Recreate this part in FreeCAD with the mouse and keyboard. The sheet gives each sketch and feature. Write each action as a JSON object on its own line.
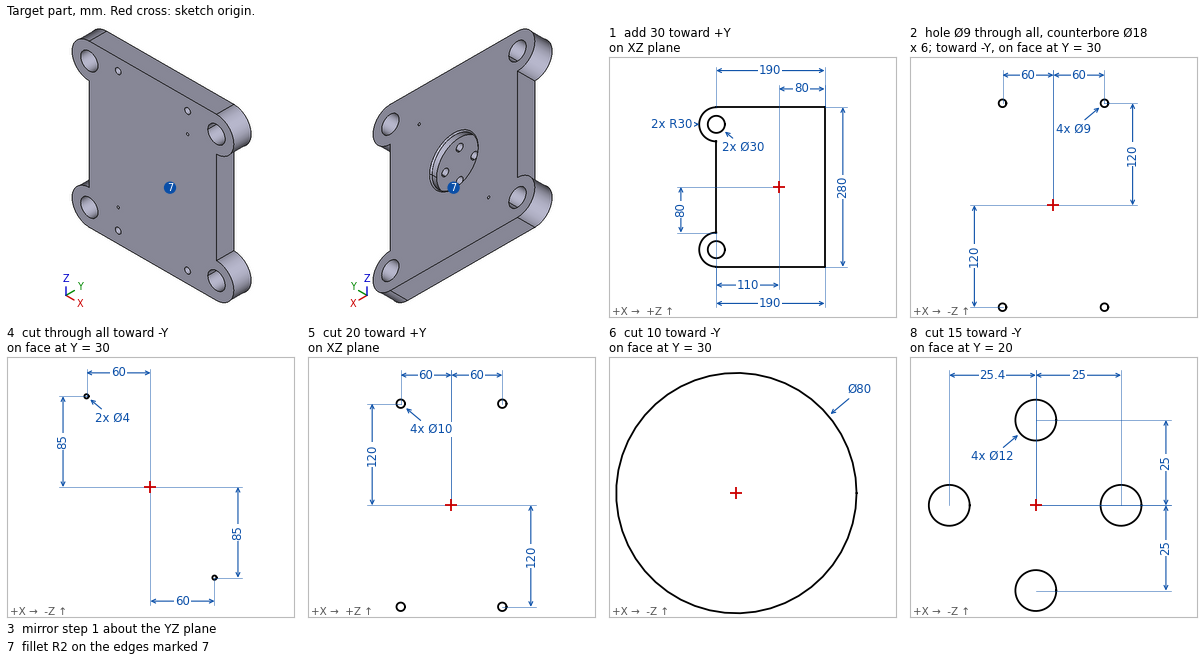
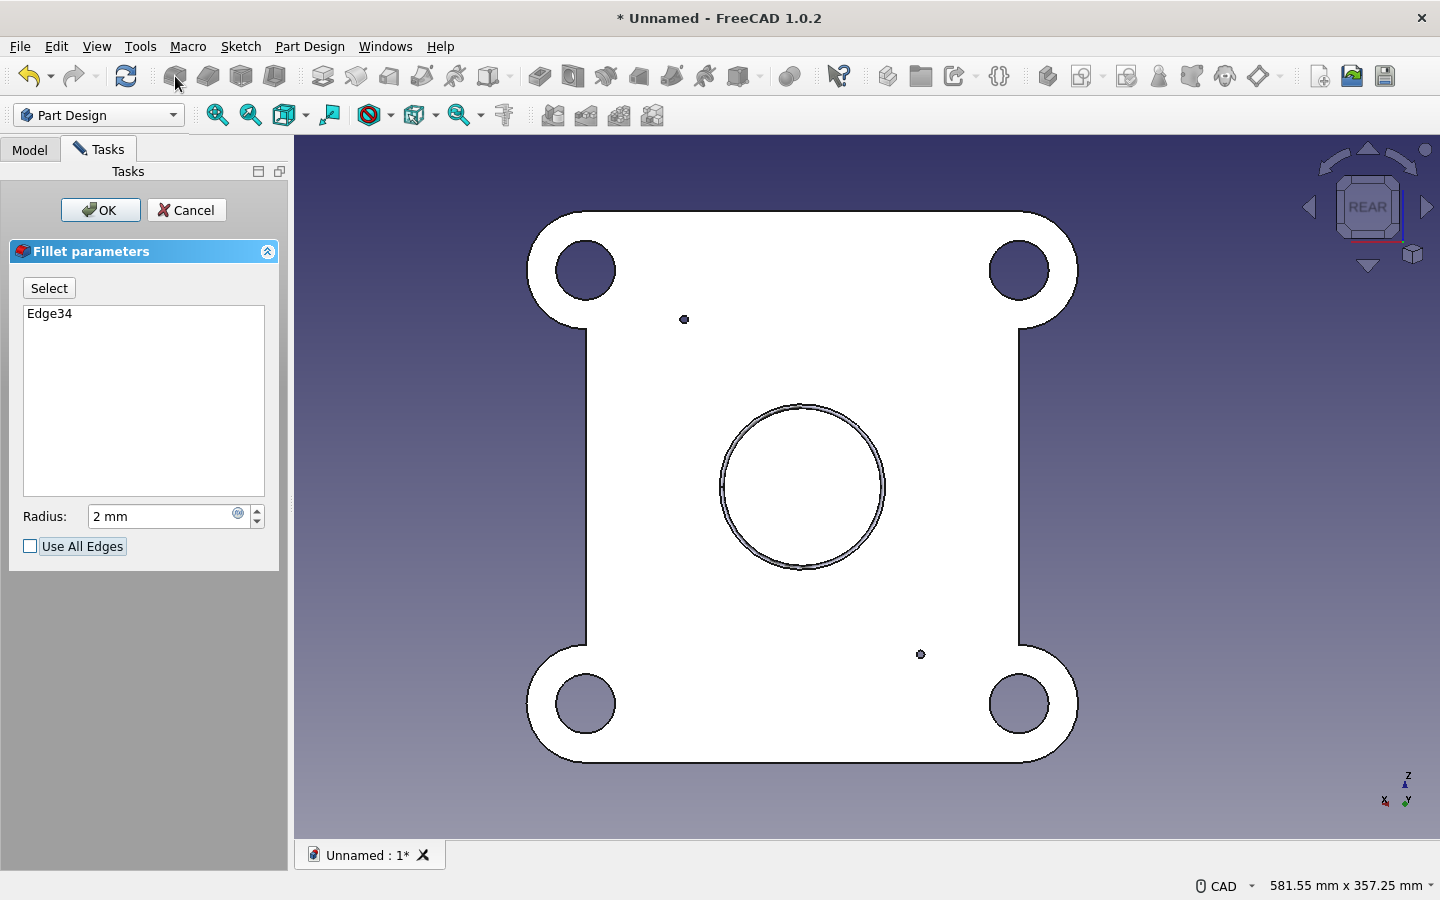
{"action": "left_click", "coordinate": [101, 210]}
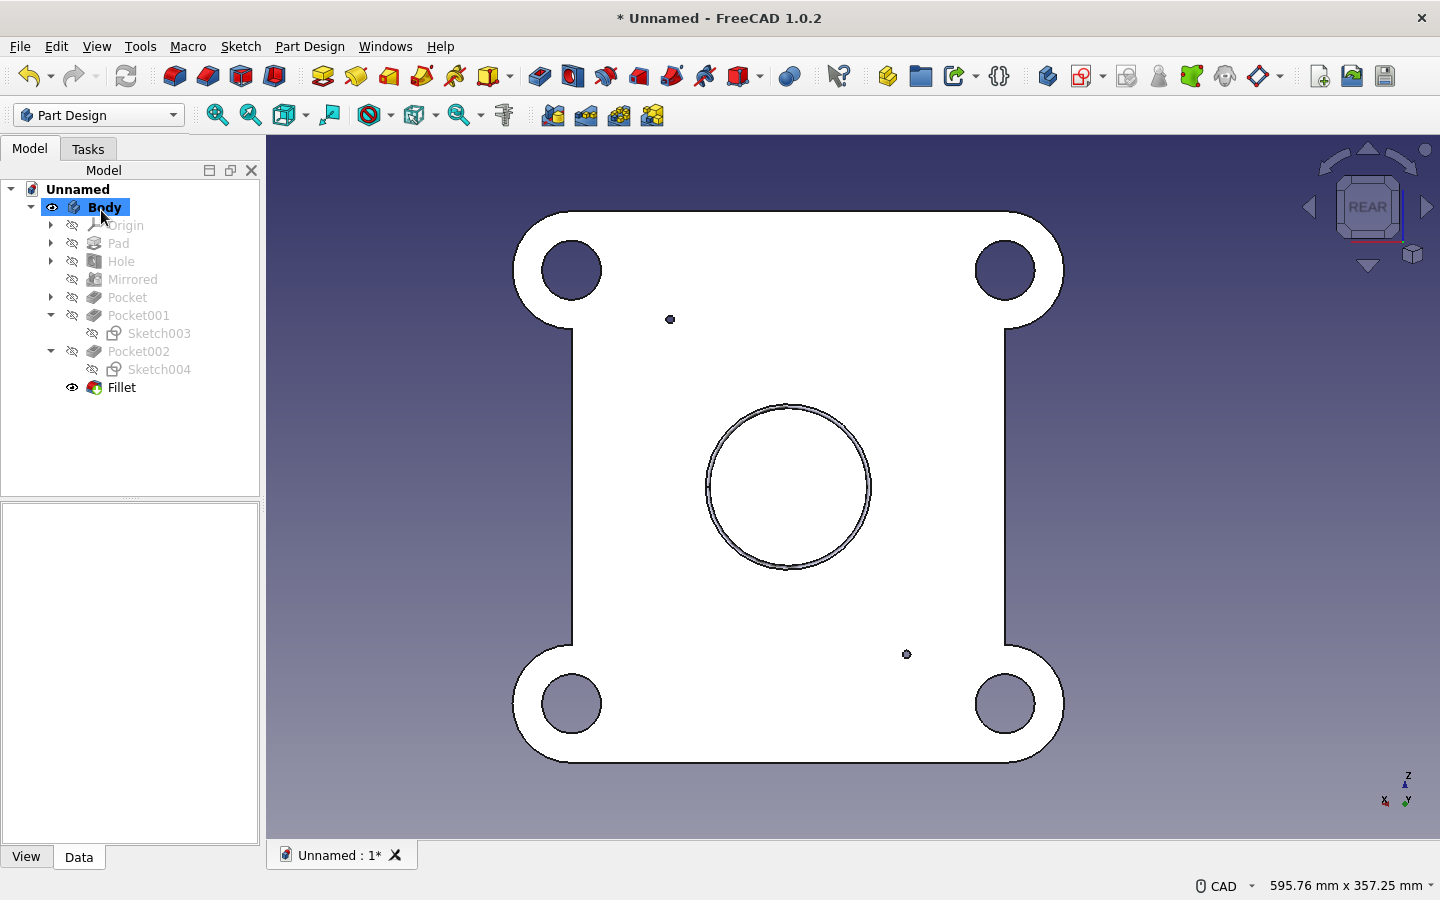
{"action": "left_click", "coordinate": [788, 486]}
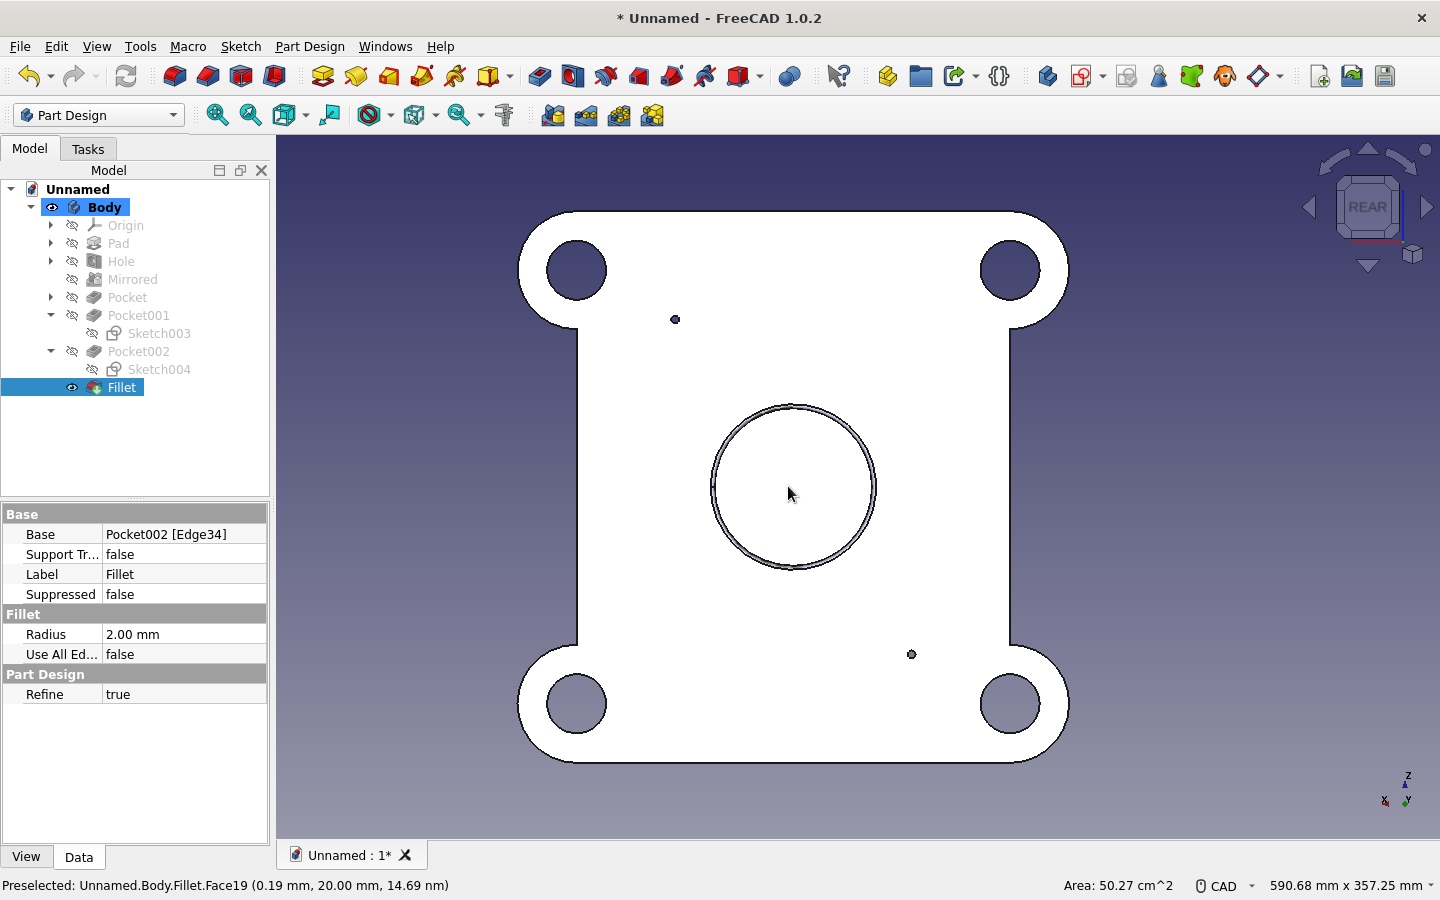
{"action": "left_click", "coordinate": [1080, 76]}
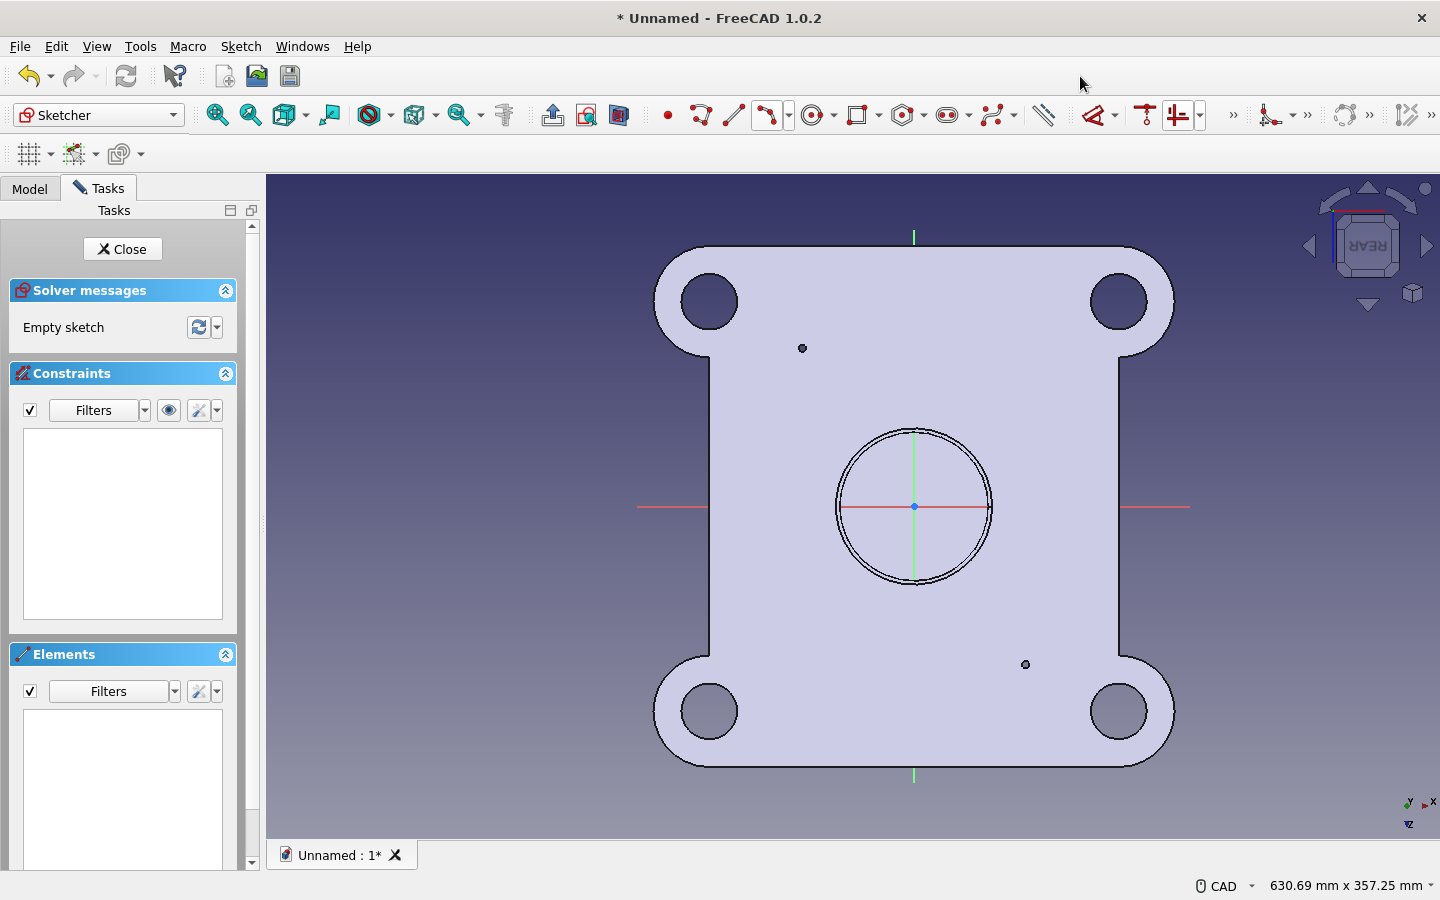
{"action": "scroll", "coordinate": [956, 506], "scroll_direction": "up", "scroll_amount": 7}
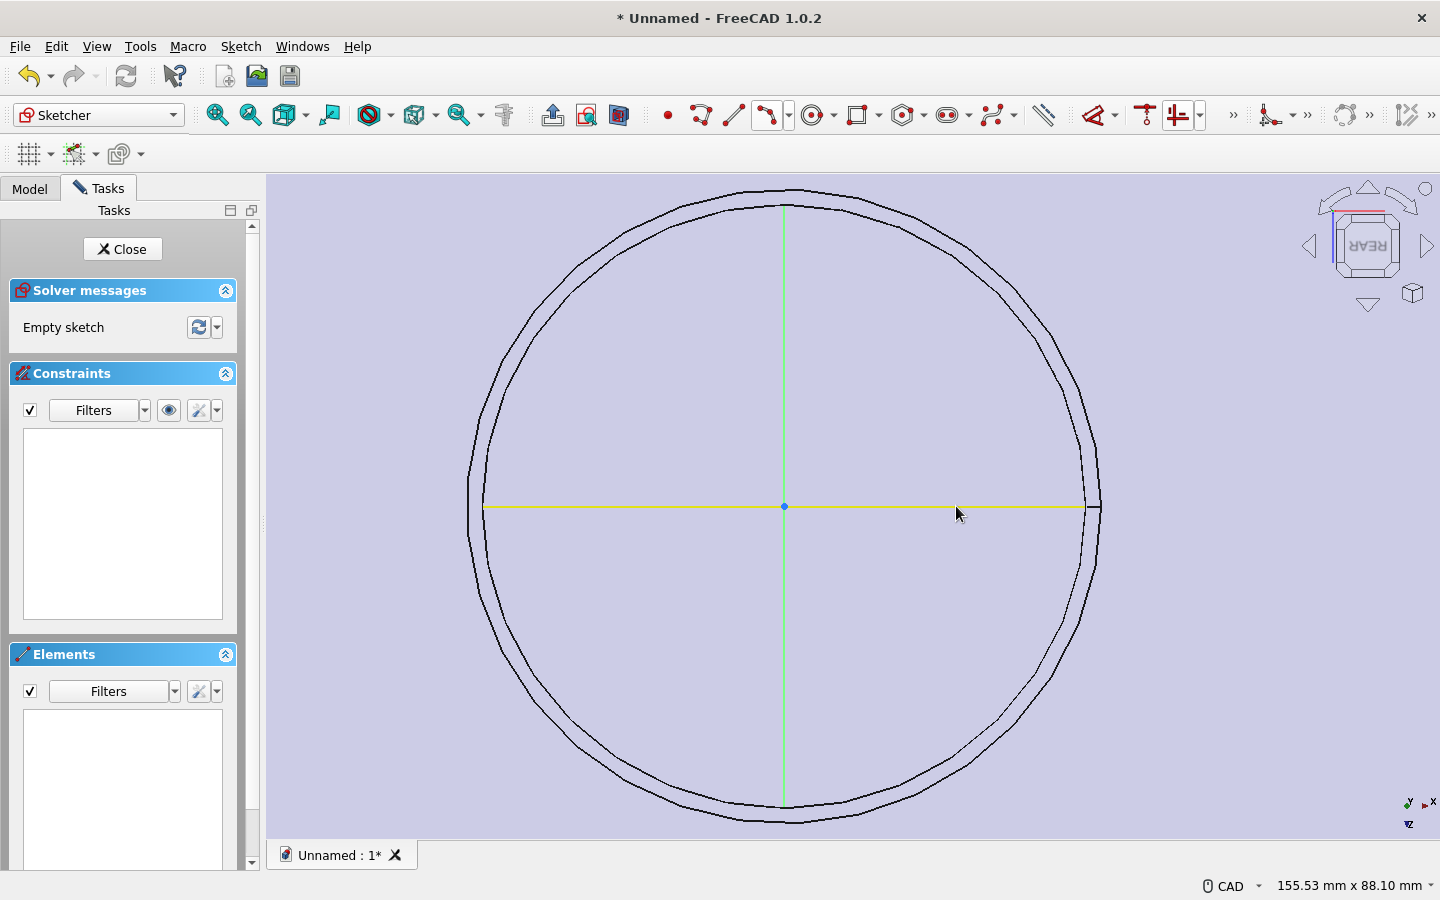
{"action": "left_click", "coordinate": [812, 116]}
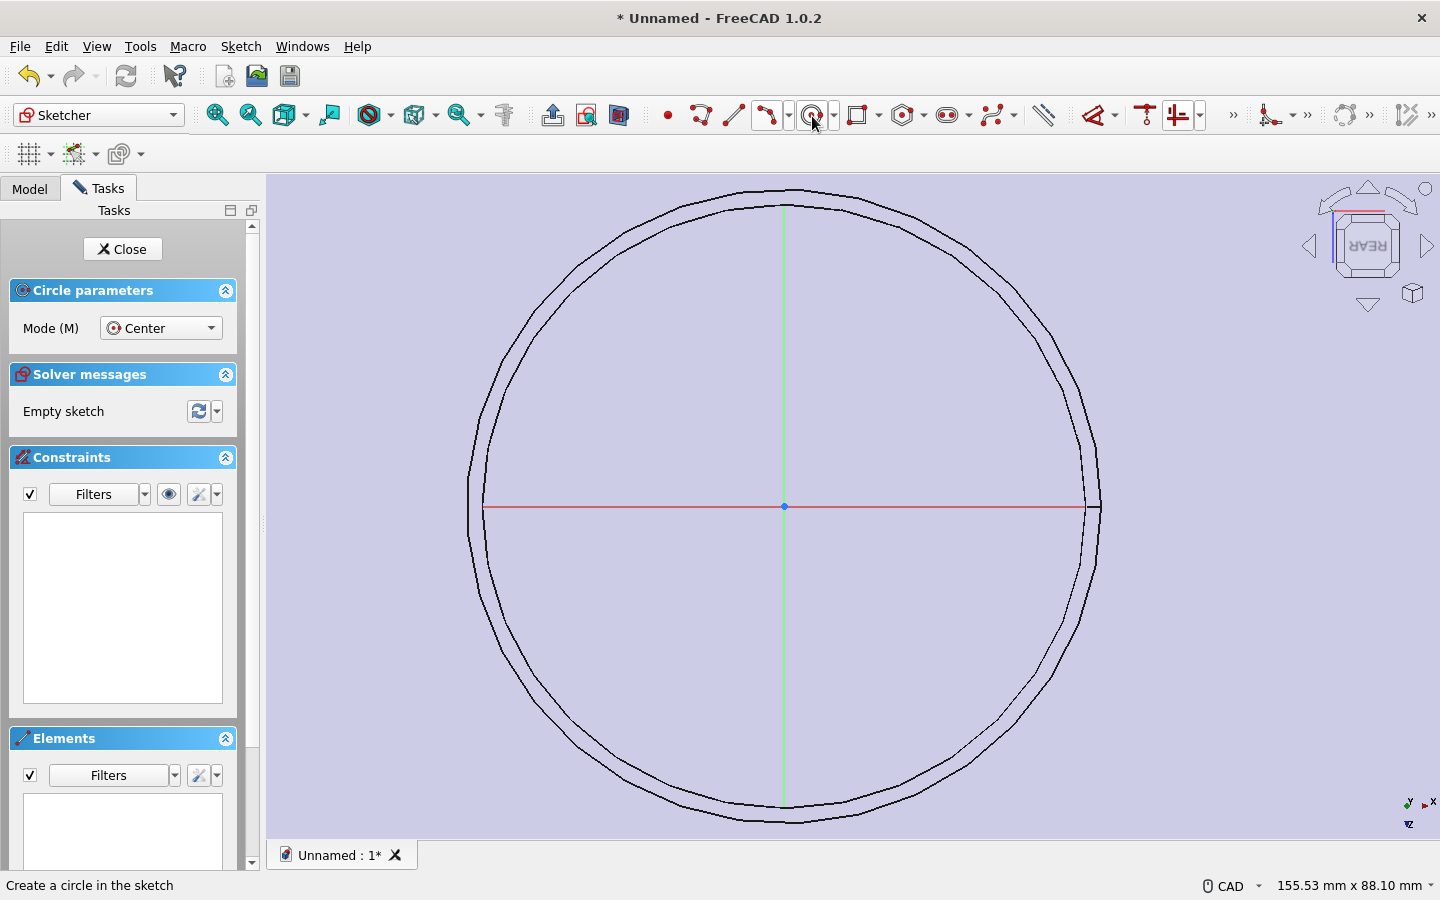
{"action": "left_click", "coordinate": [784, 318]}
{"action": "mouse_move", "coordinate": [816, 286]}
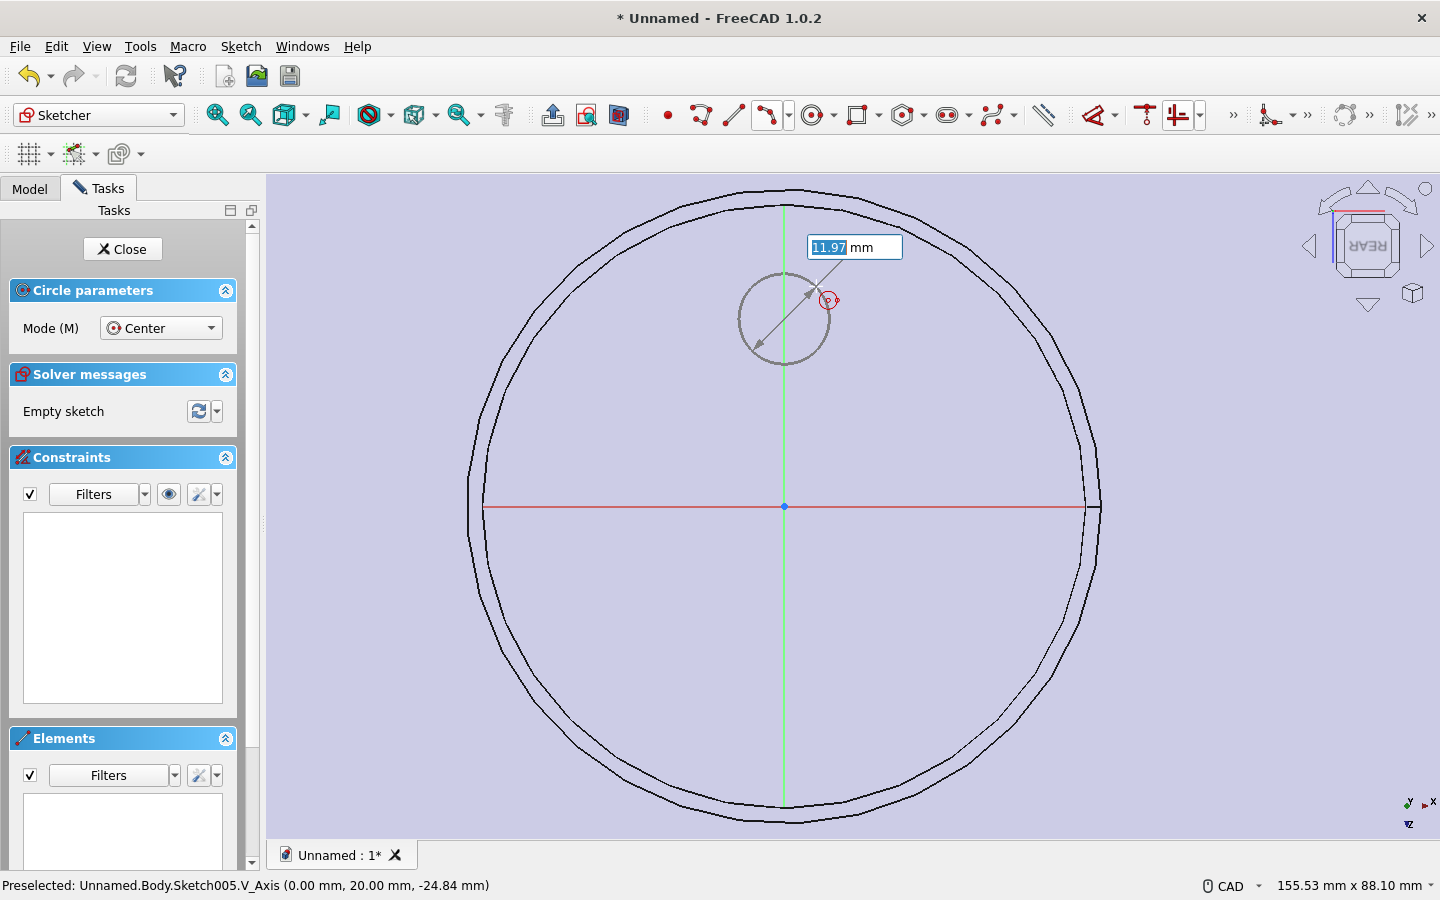
{"action": "type", "text": "12"}
{"action": "key", "text": "Return"}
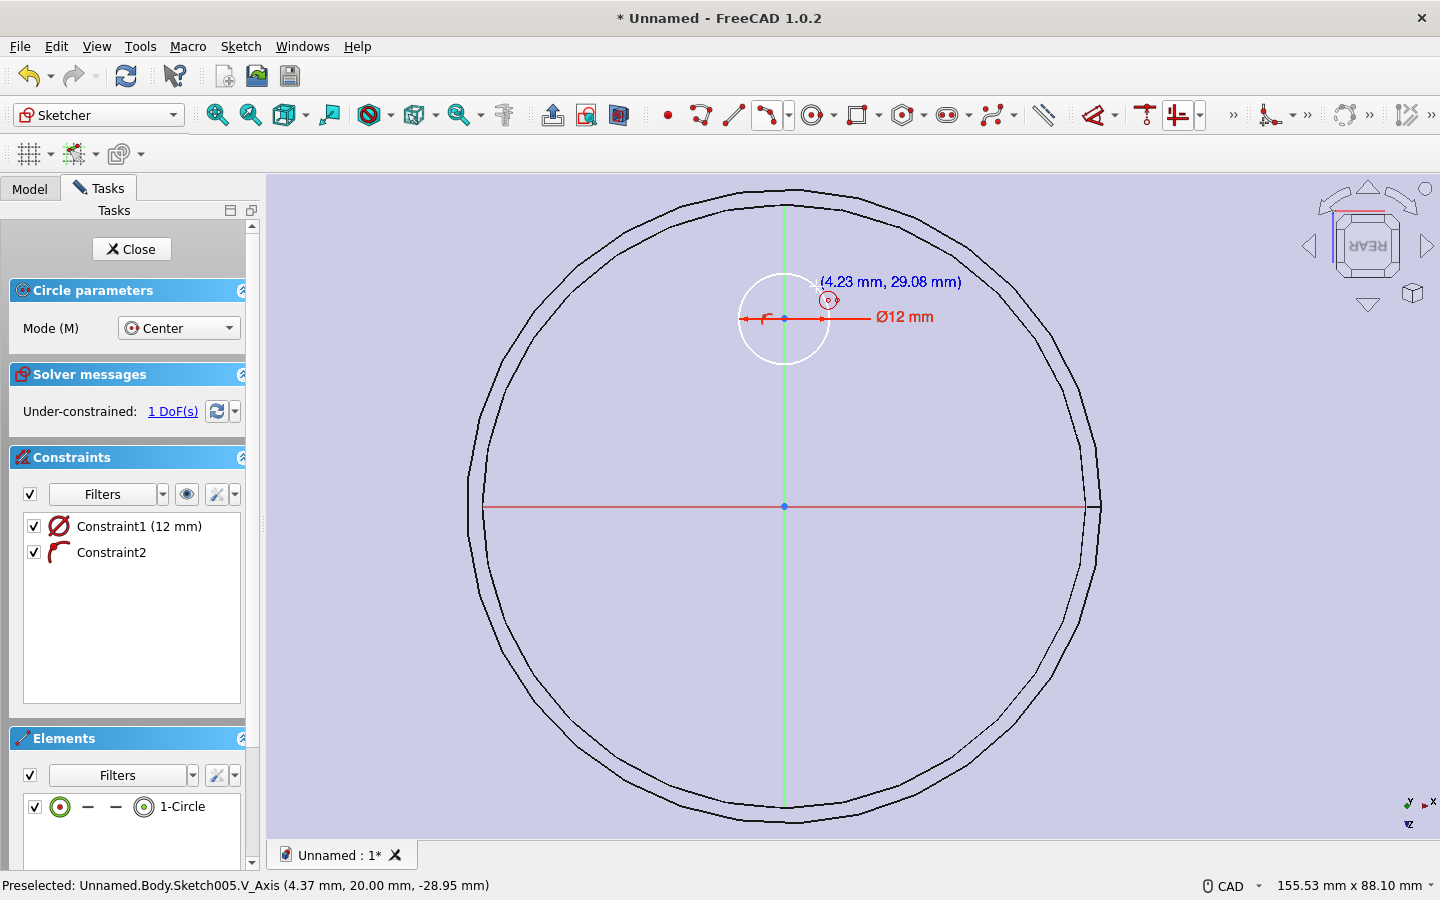
{"action": "left_click", "coordinate": [592, 506]}
{"action": "mouse_move", "coordinate": [624, 474]}